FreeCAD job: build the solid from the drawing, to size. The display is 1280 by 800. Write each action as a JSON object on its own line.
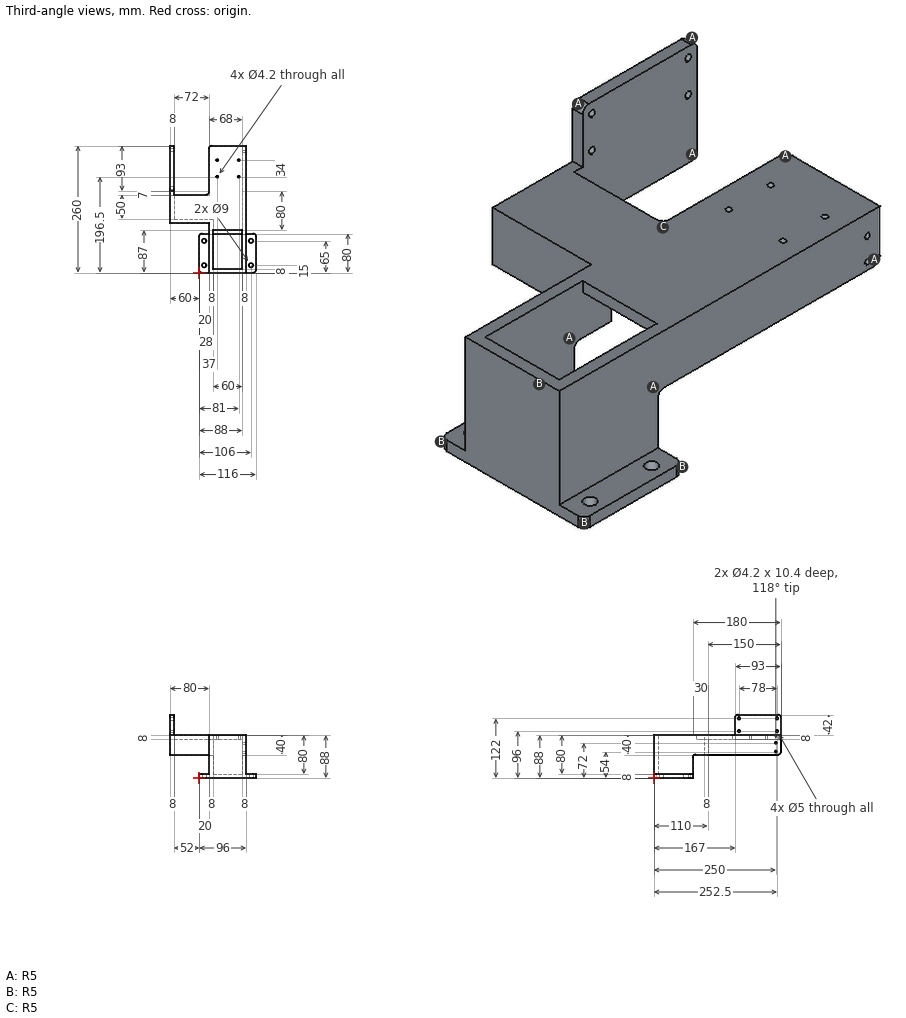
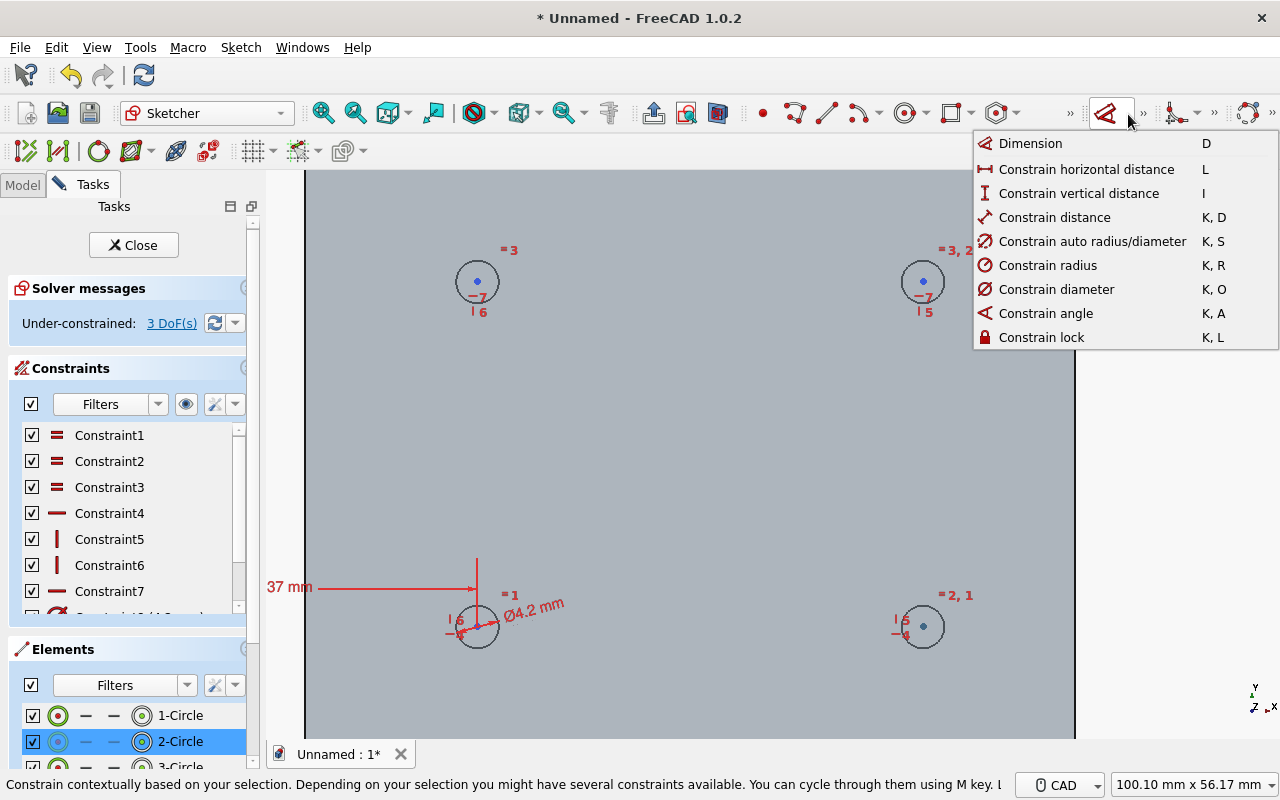
{"action": "left_click", "coordinate": [1126, 169]}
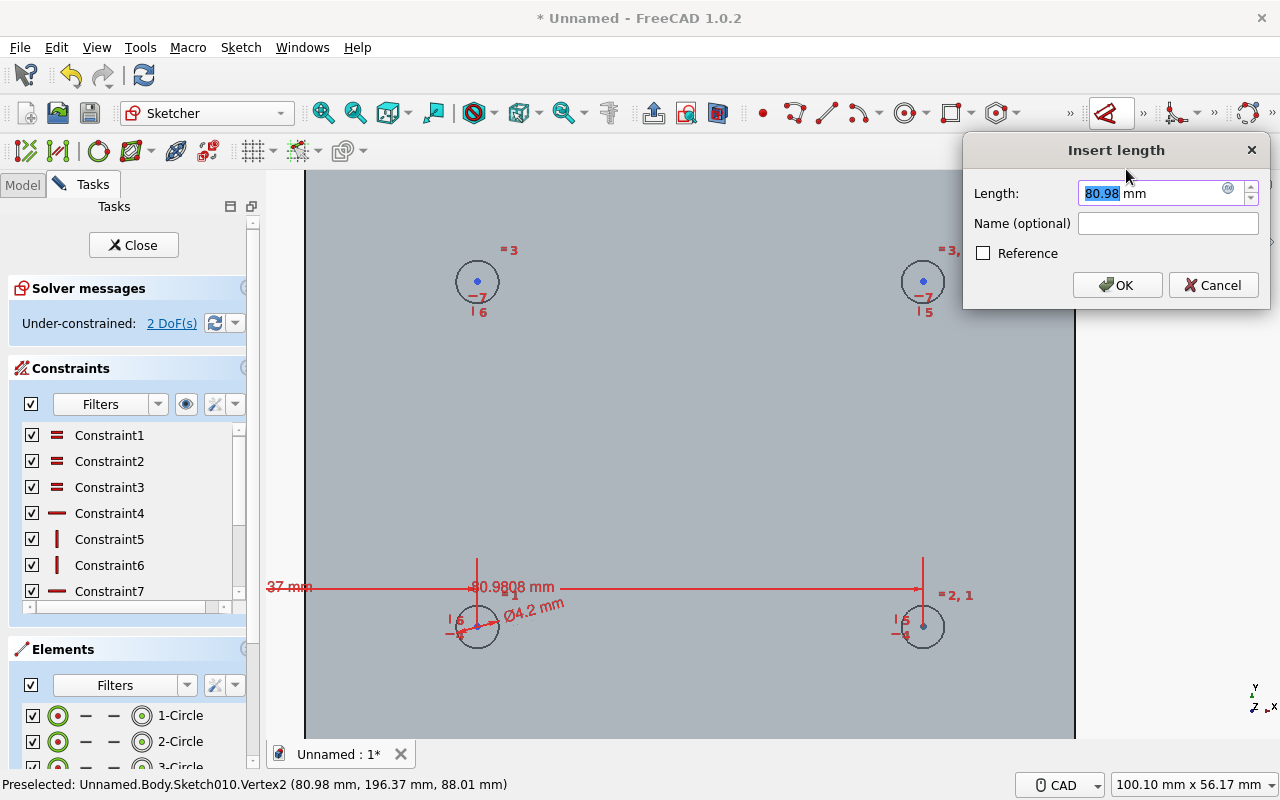
{"action": "type", "text": "81"}
{"action": "key", "text": "Return"}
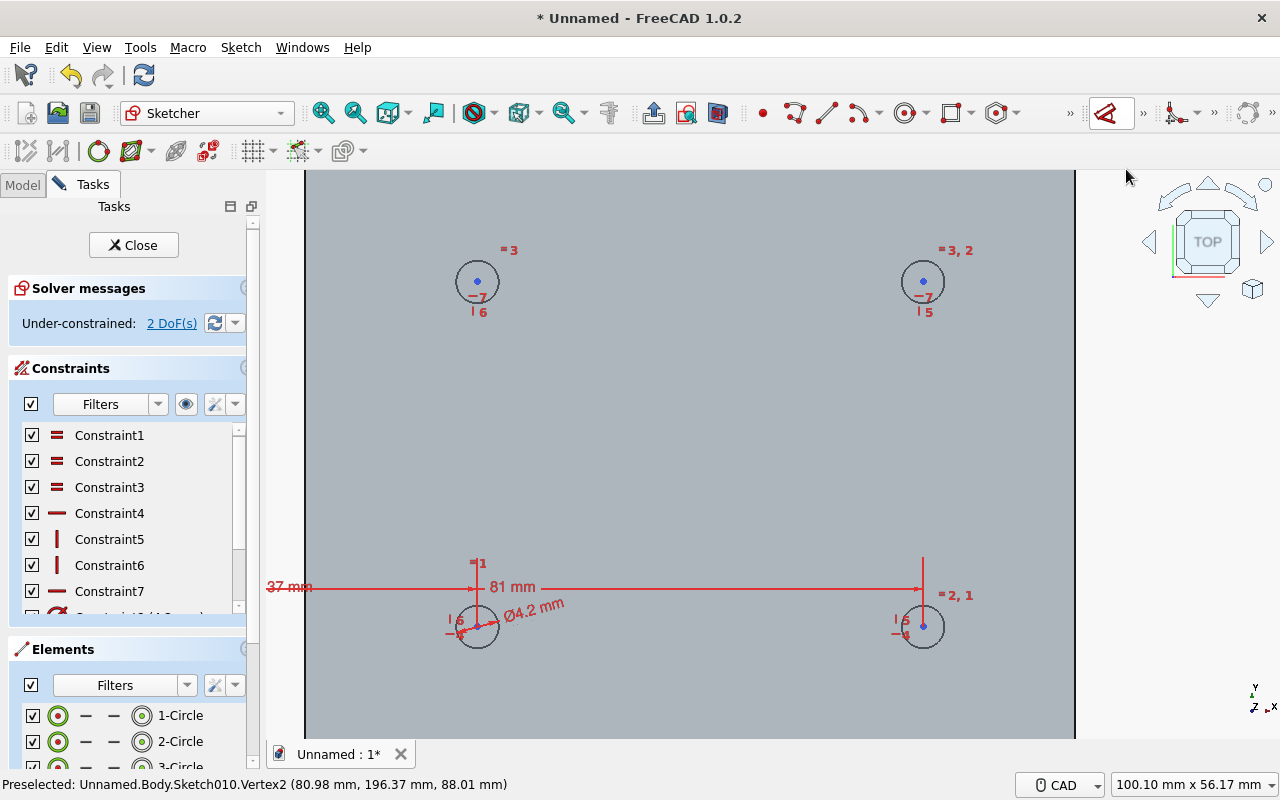
{"action": "left_click", "coordinate": [923, 627]}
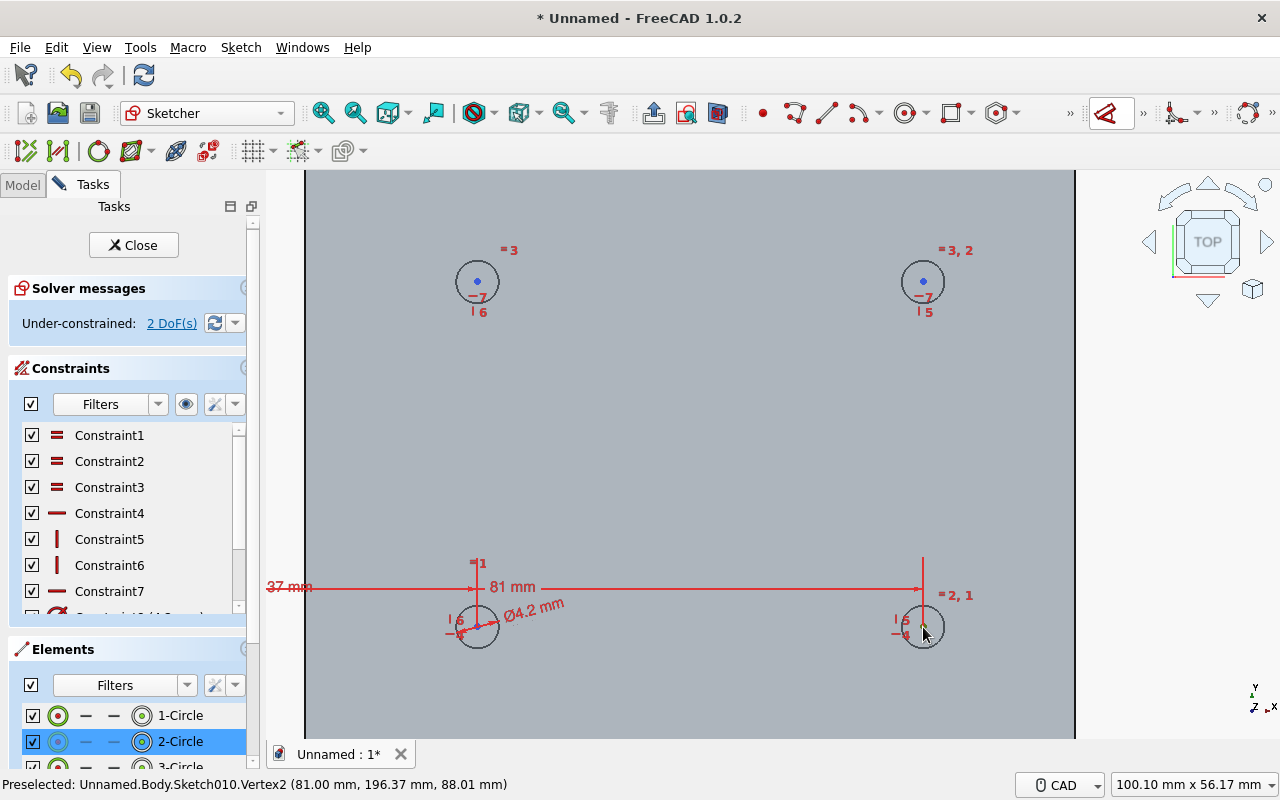
{"action": "left_click", "coordinate": [923, 282]}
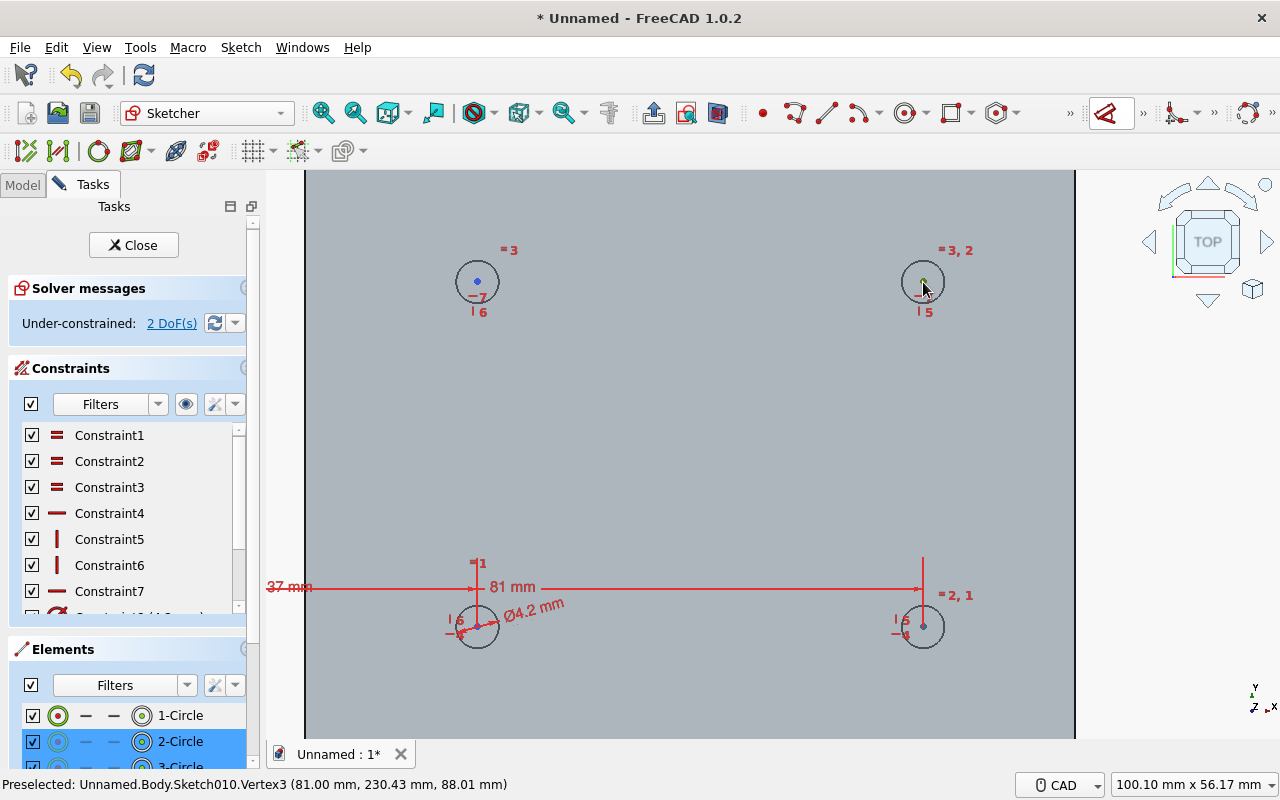
{"action": "left_click", "coordinate": [1128, 114]}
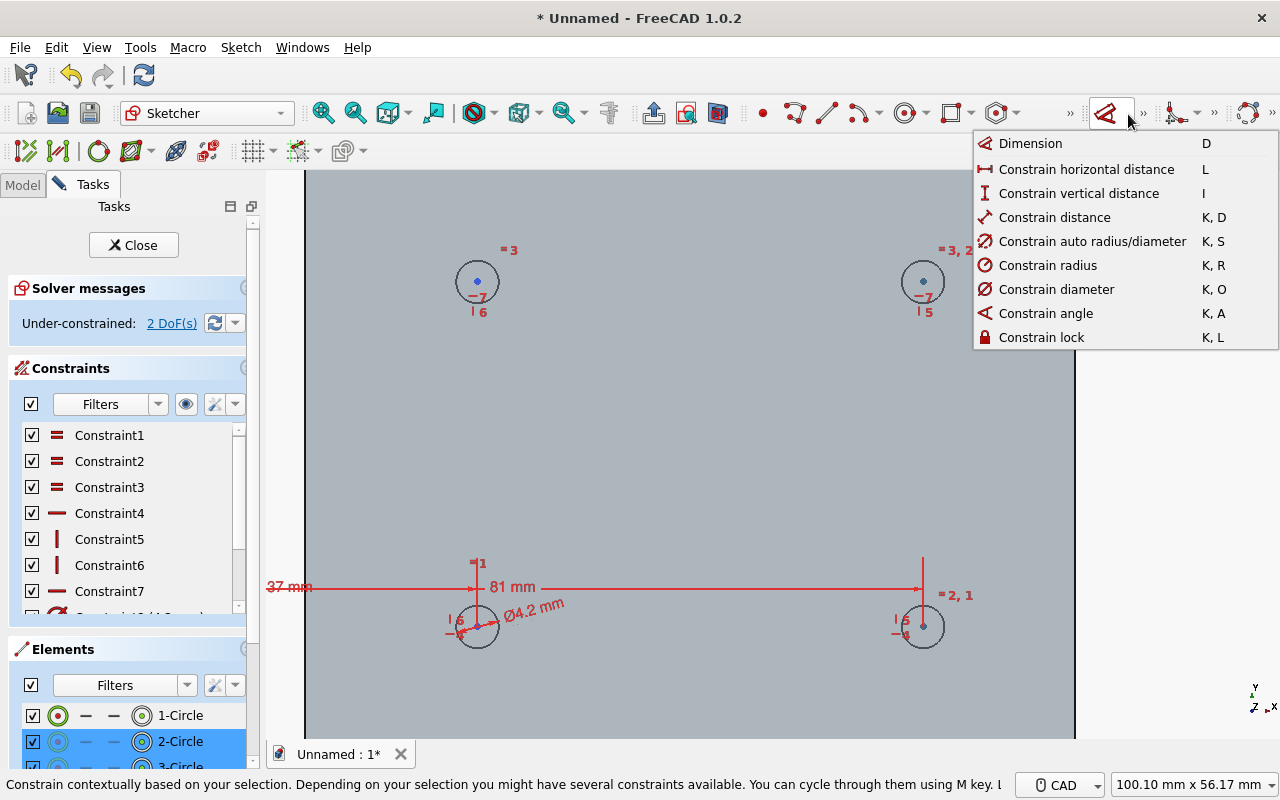
{"action": "left_click", "coordinate": [1126, 193]}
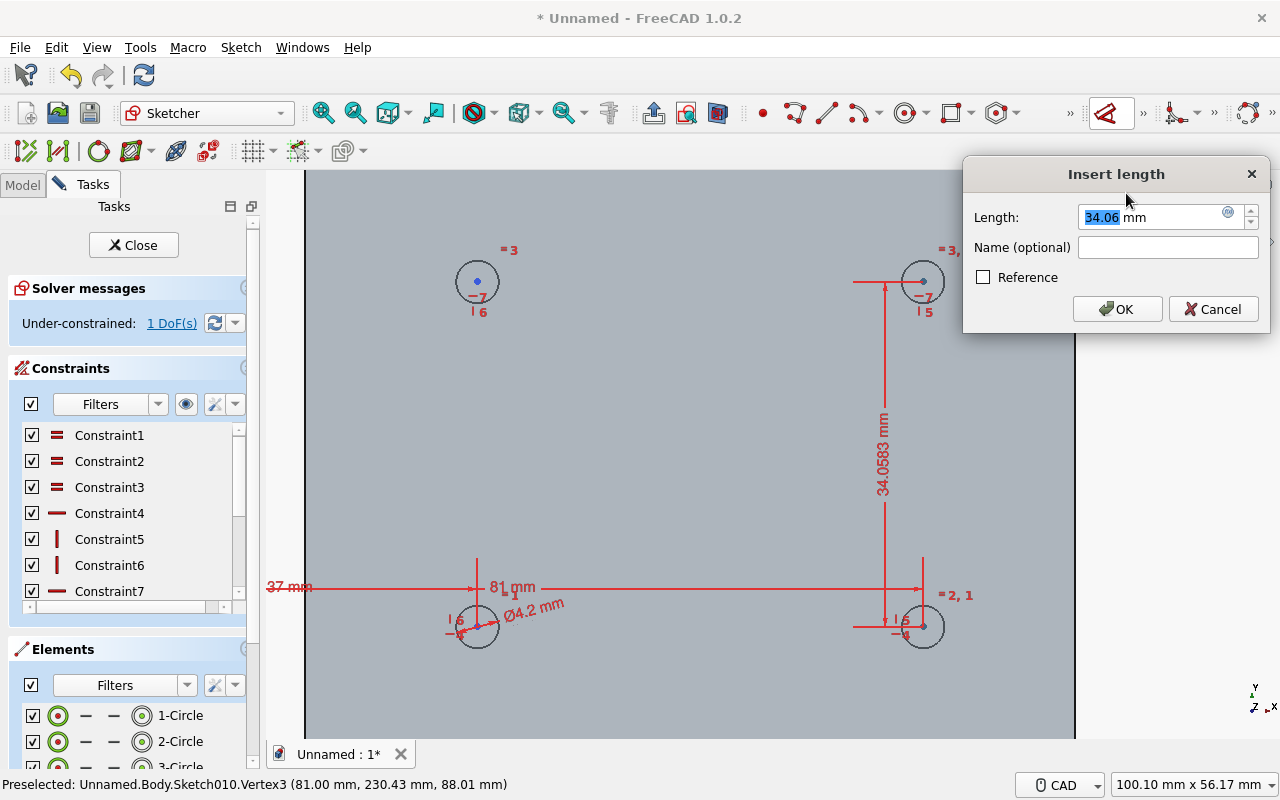
{"action": "type", "text": "34"}
{"action": "key", "text": "Return"}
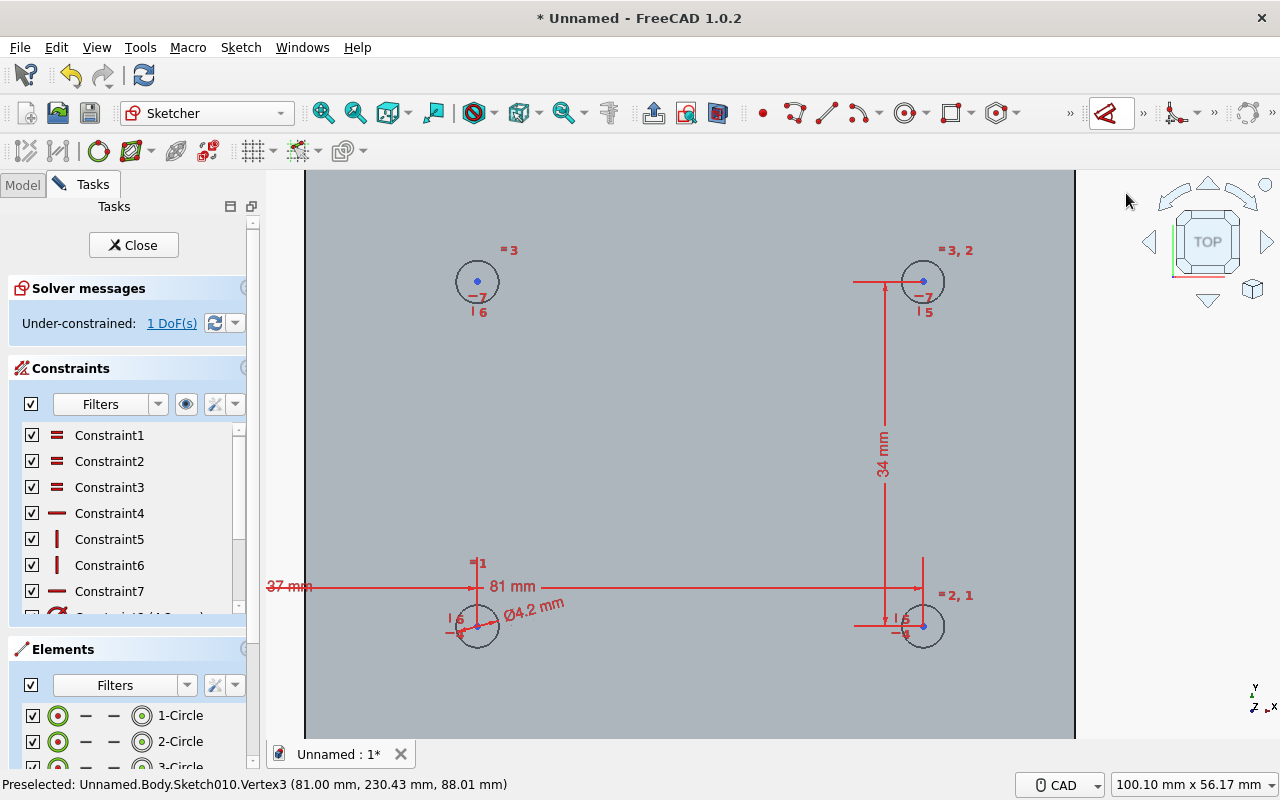
{"action": "left_click", "coordinate": [477, 626]}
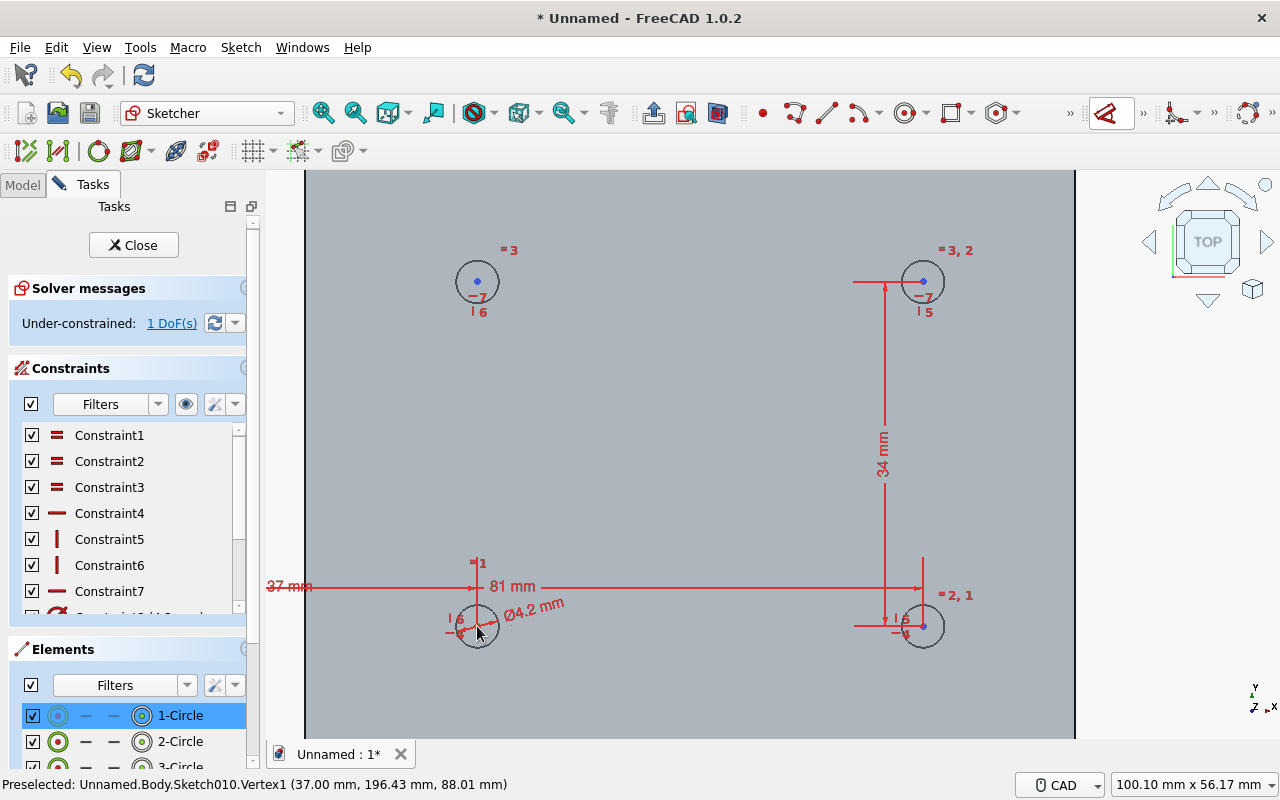
{"action": "left_click", "coordinate": [1128, 114]}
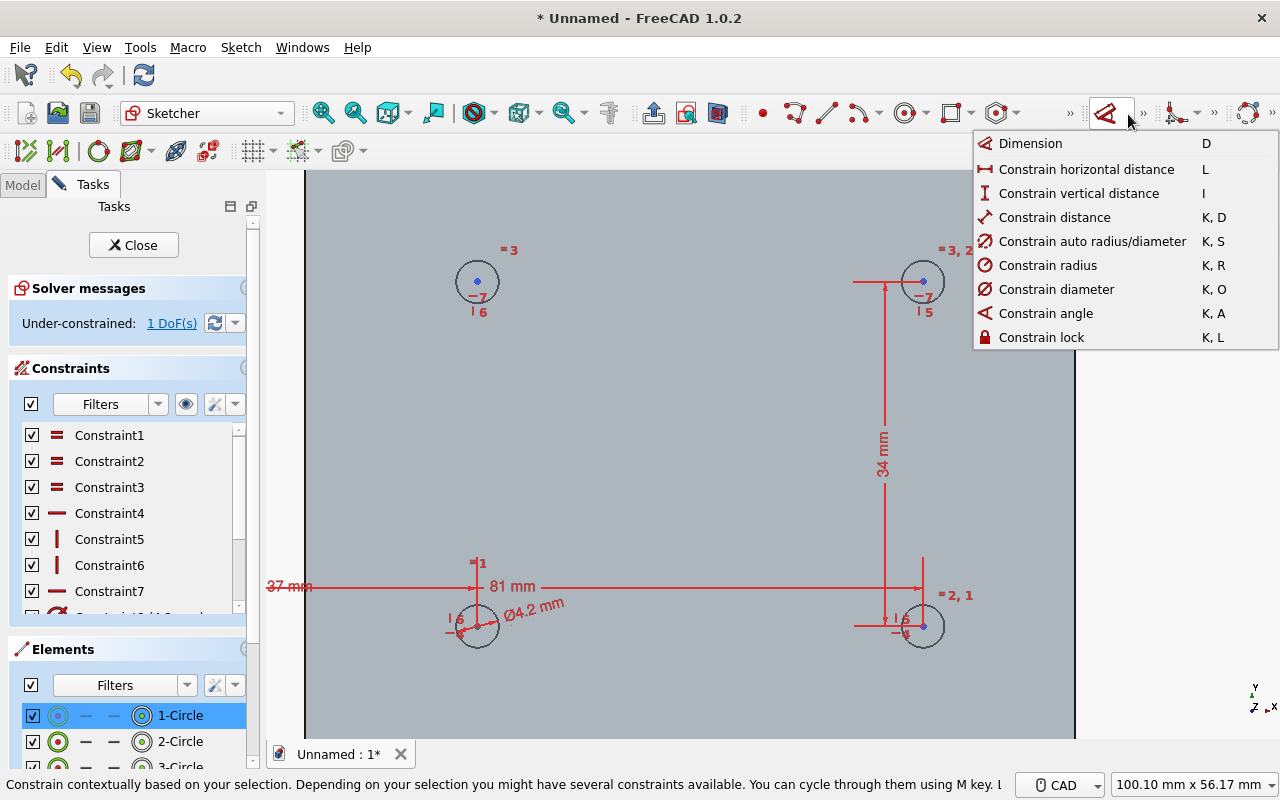
{"action": "left_click", "coordinate": [1126, 193]}